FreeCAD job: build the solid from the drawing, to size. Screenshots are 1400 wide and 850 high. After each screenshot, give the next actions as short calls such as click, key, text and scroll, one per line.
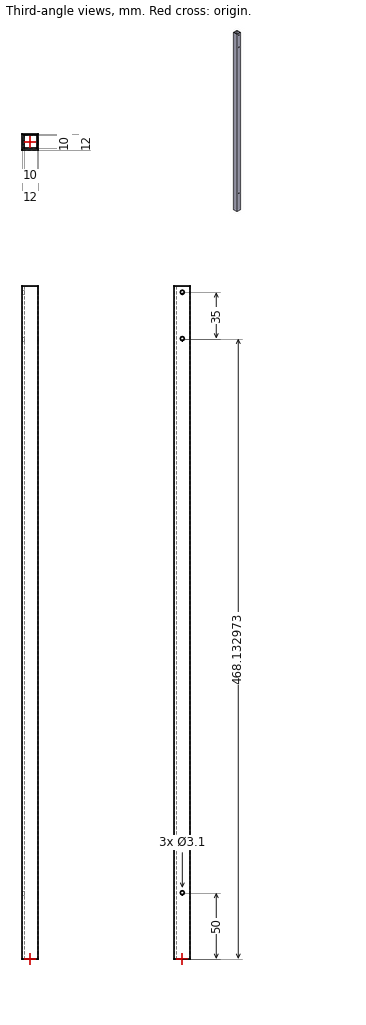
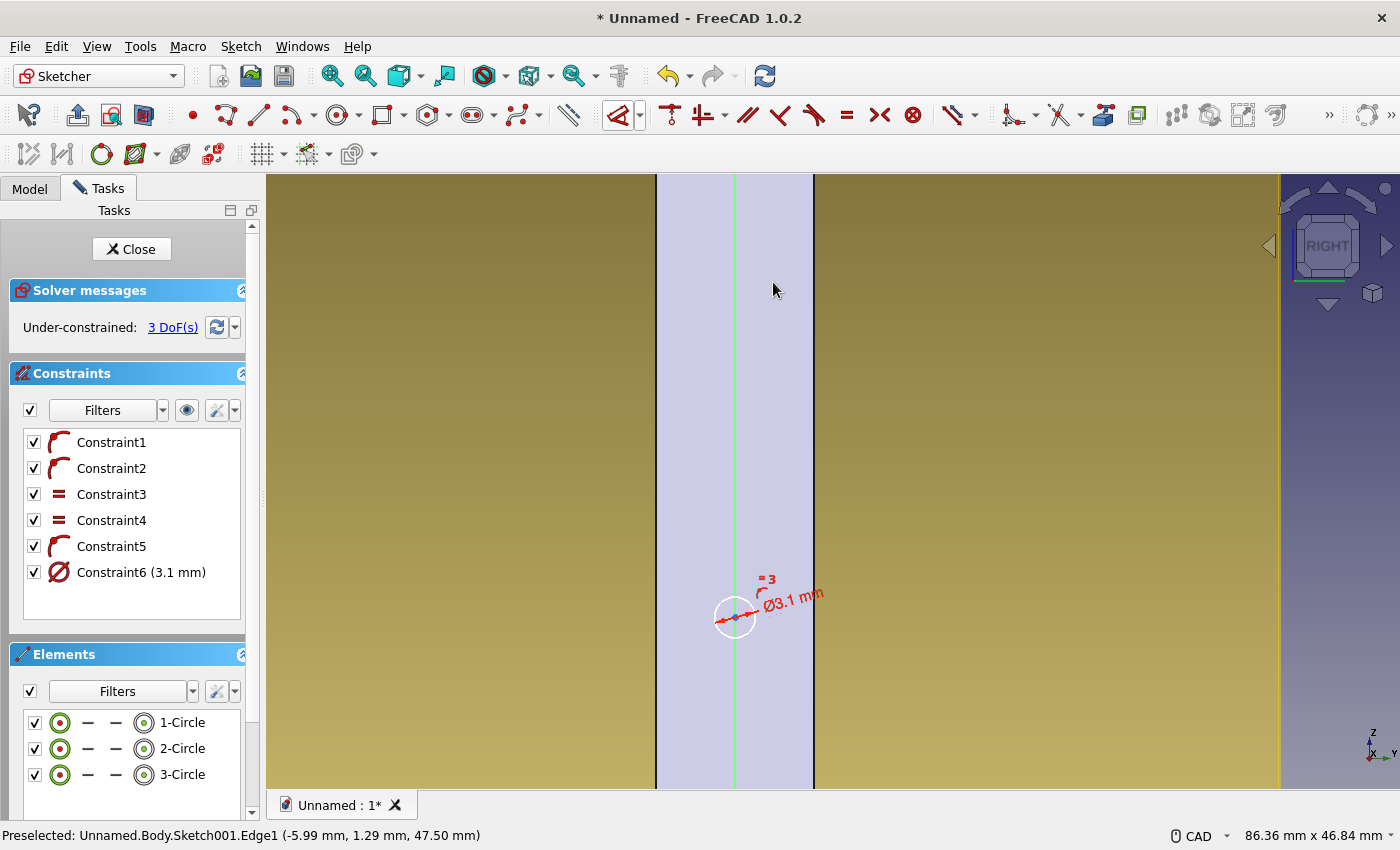
scroll(766, 646, down, 14)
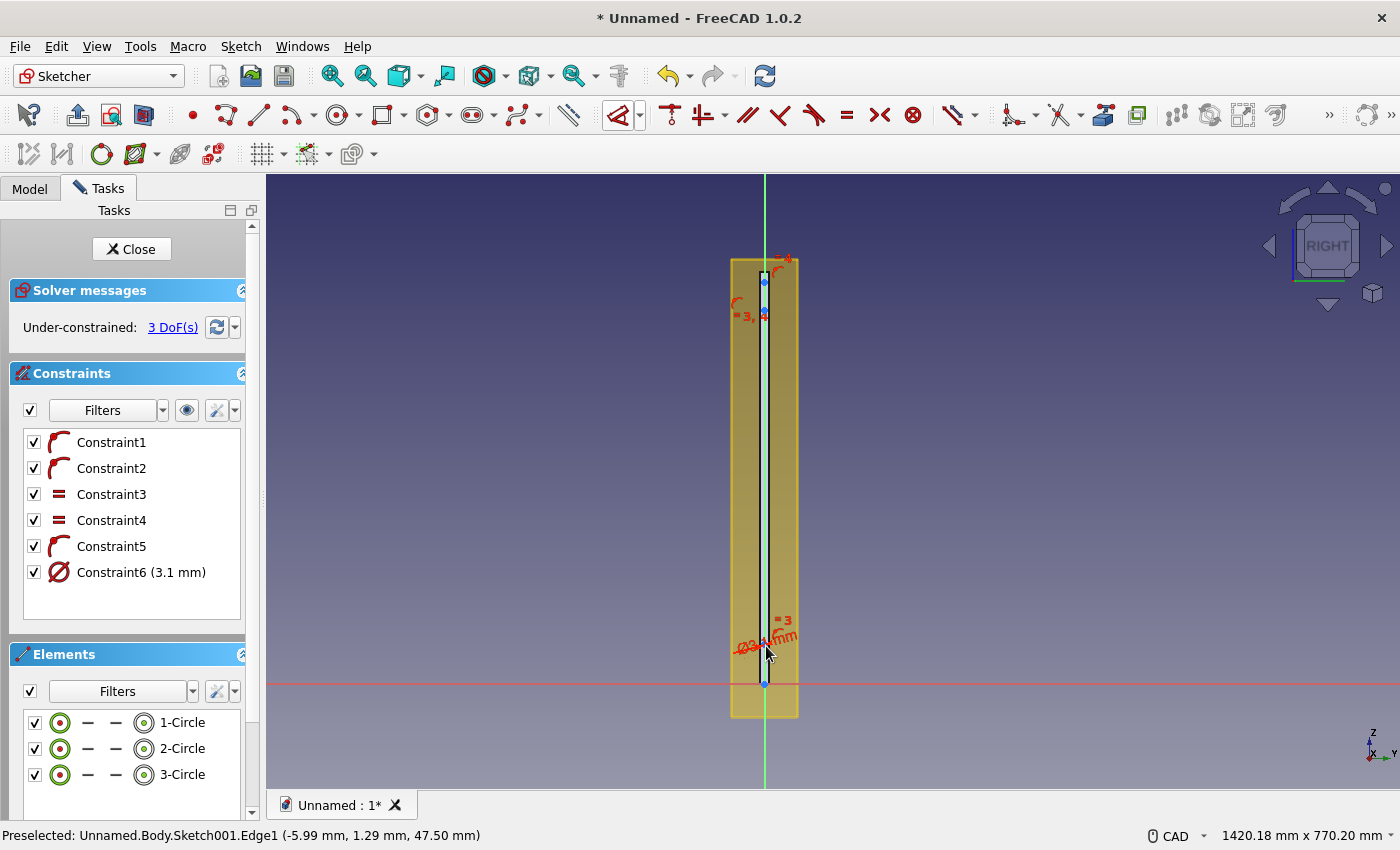
click(765, 645)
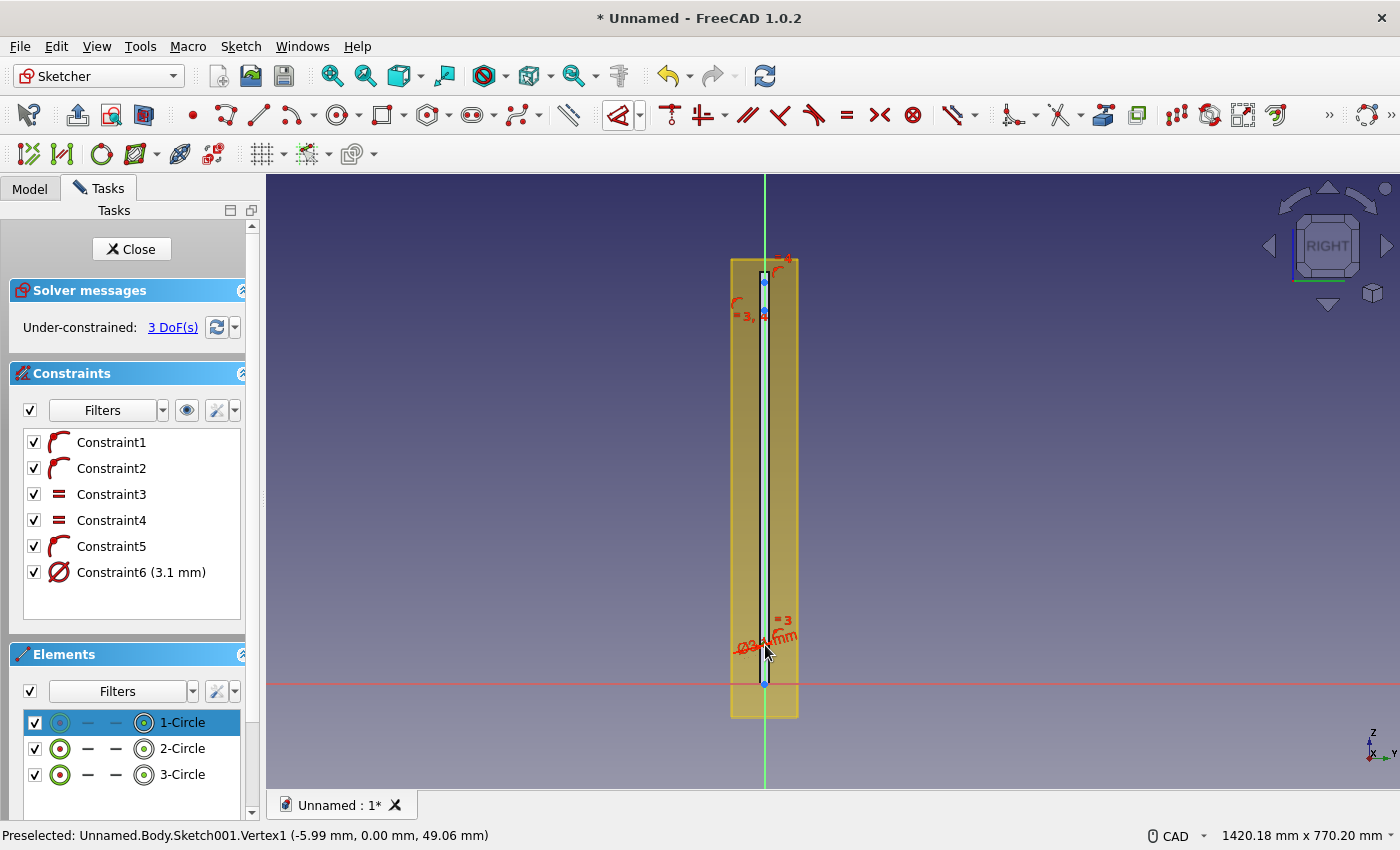
click(640, 116)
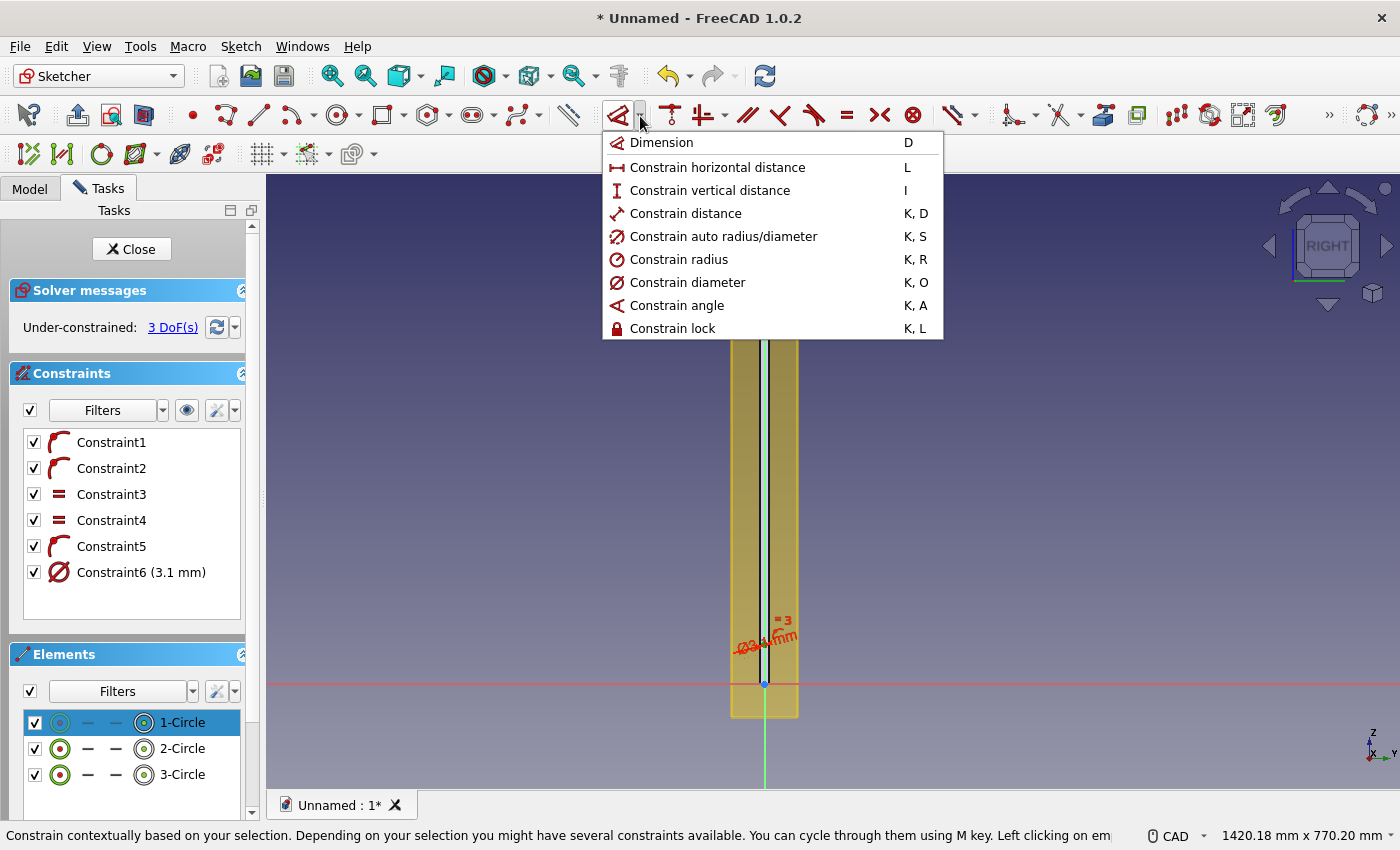
click(773, 190)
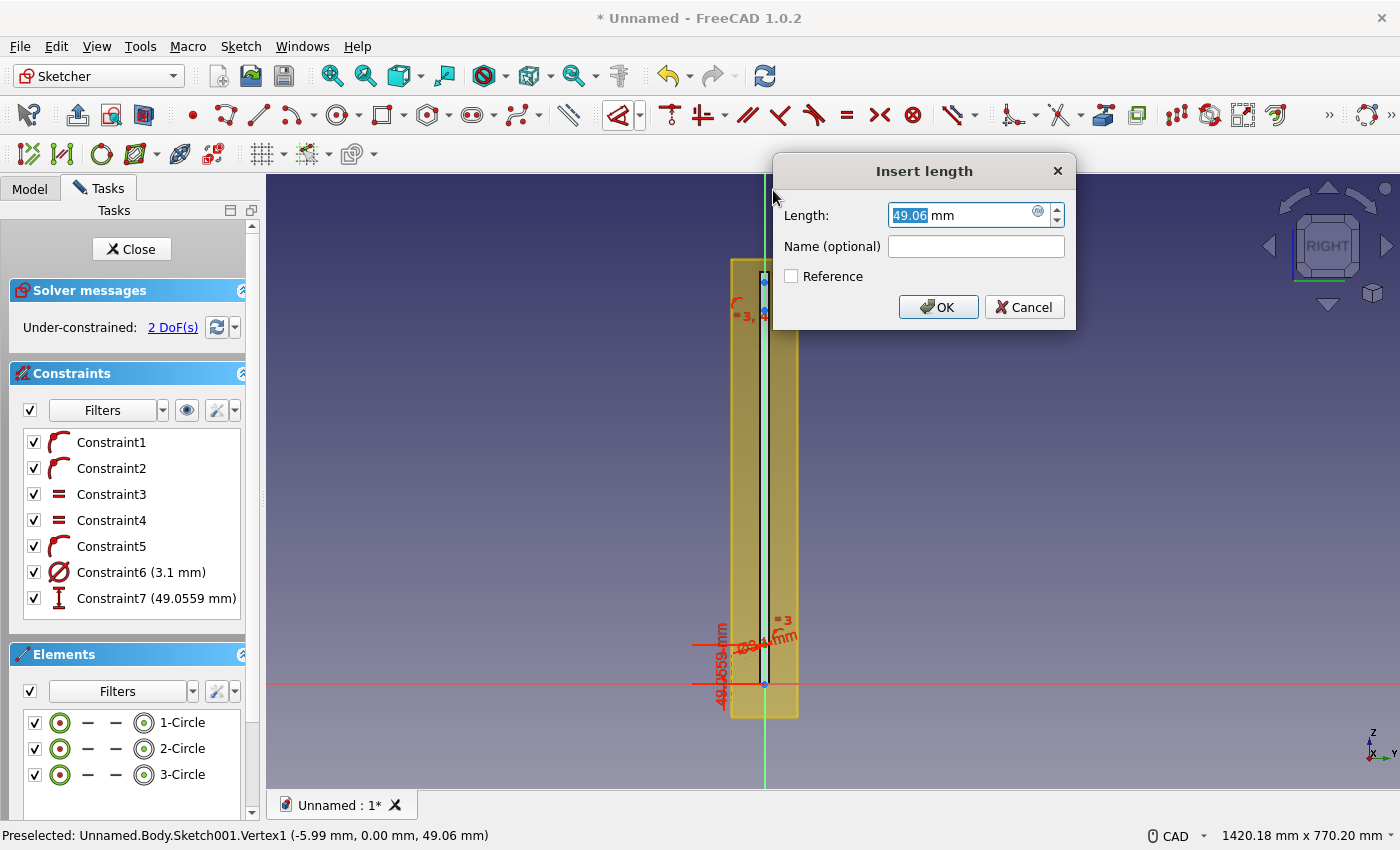
text(50)
key(Return)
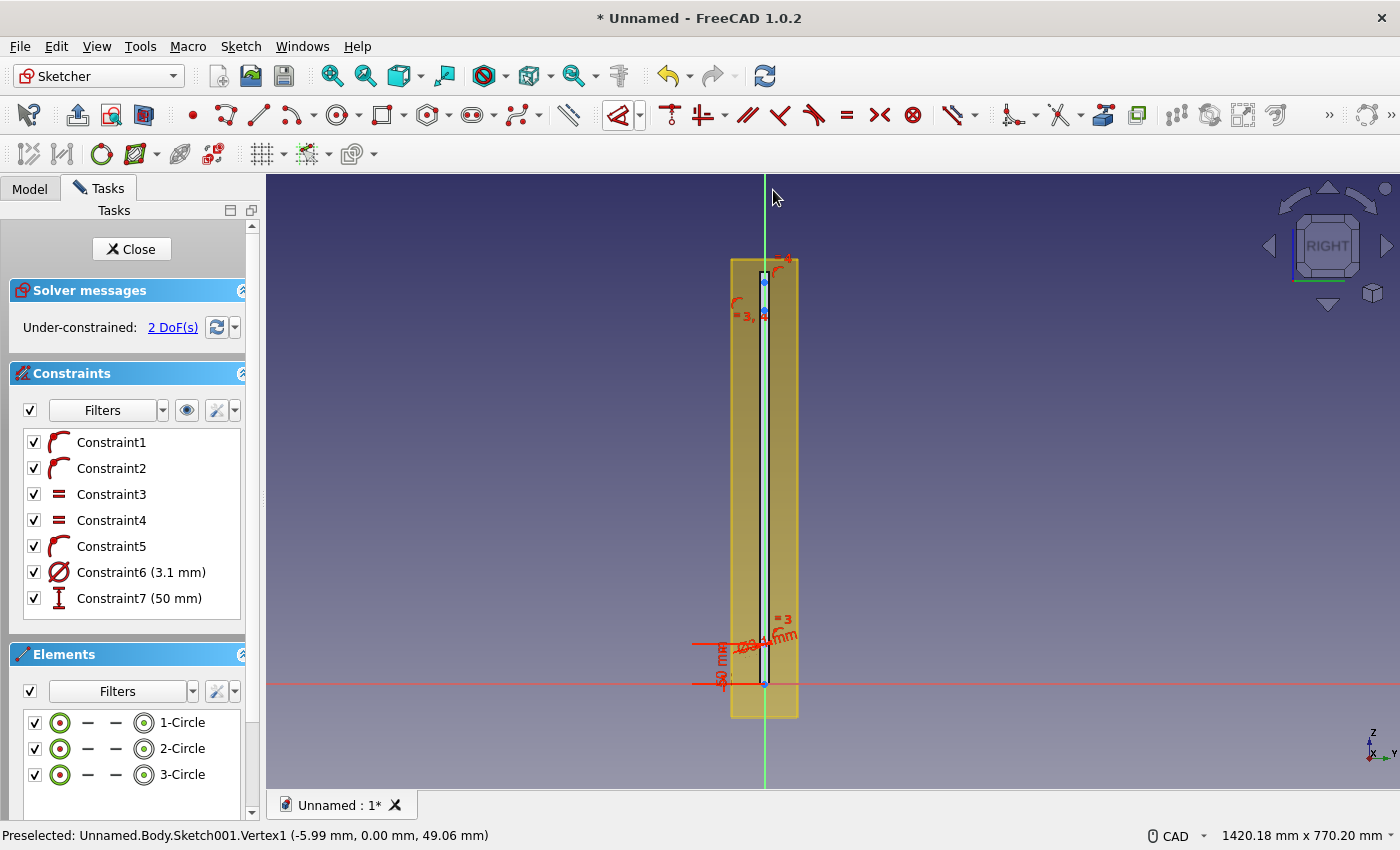
scroll(765, 311, up, 2)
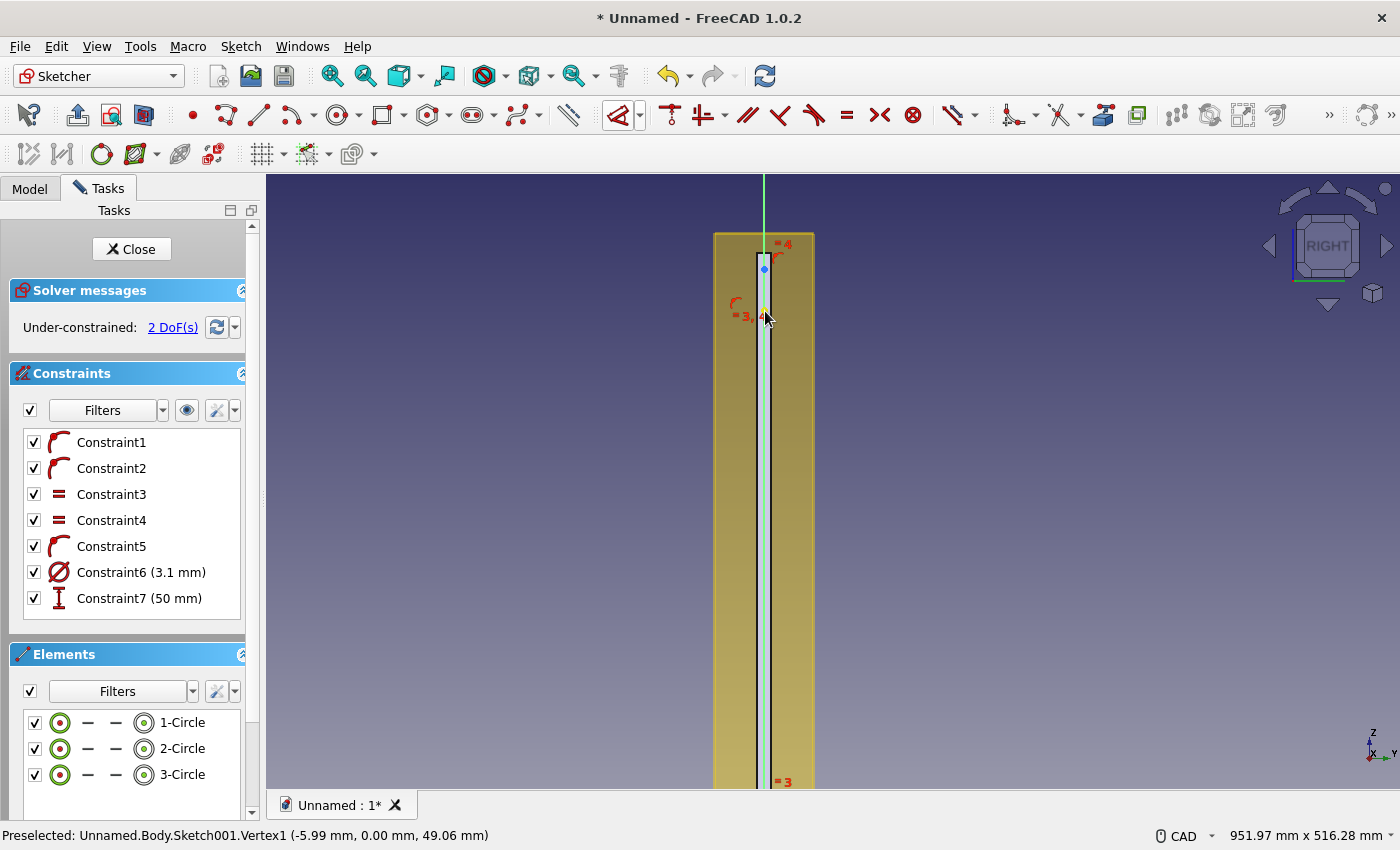
click(764, 311)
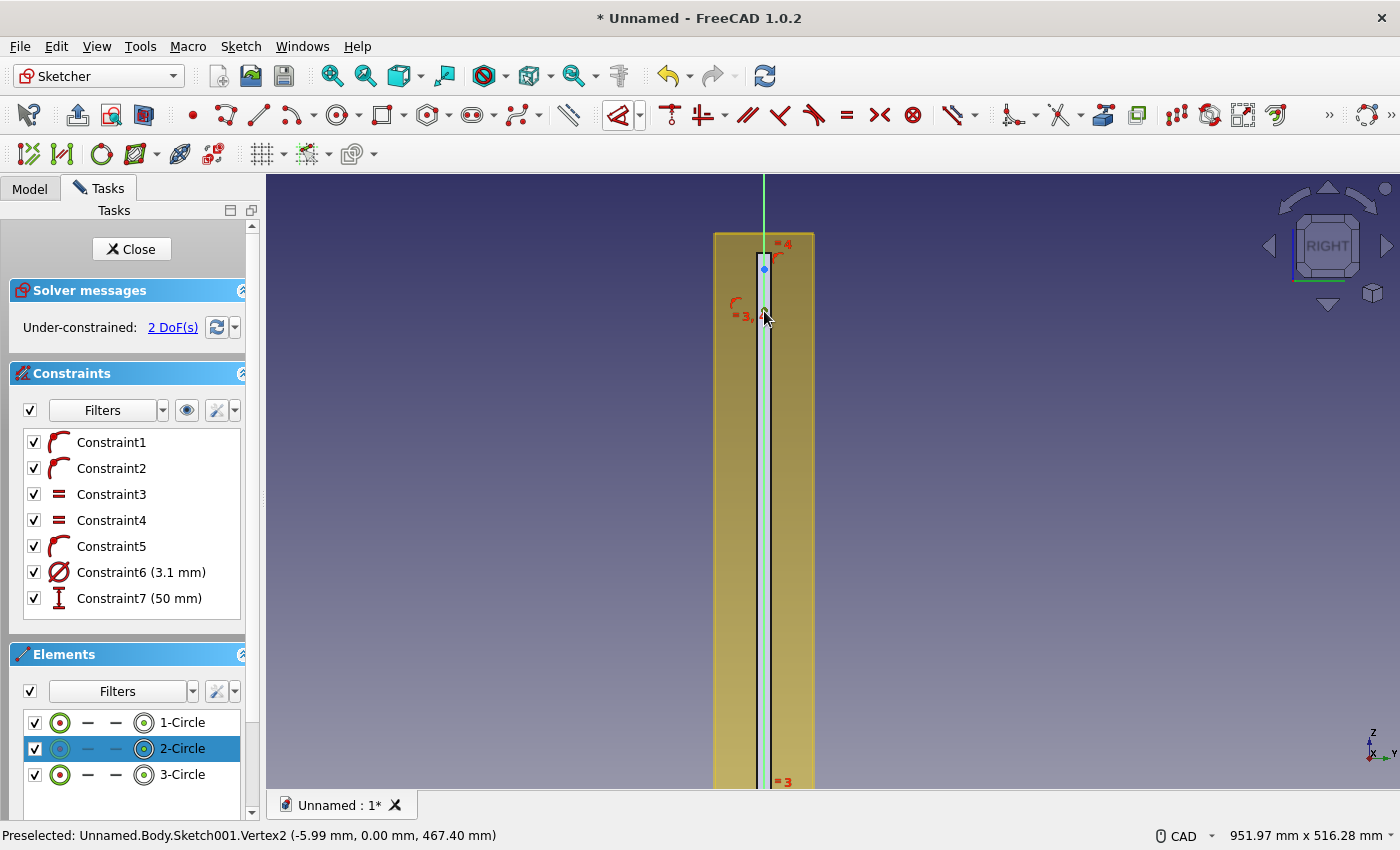
click(764, 269)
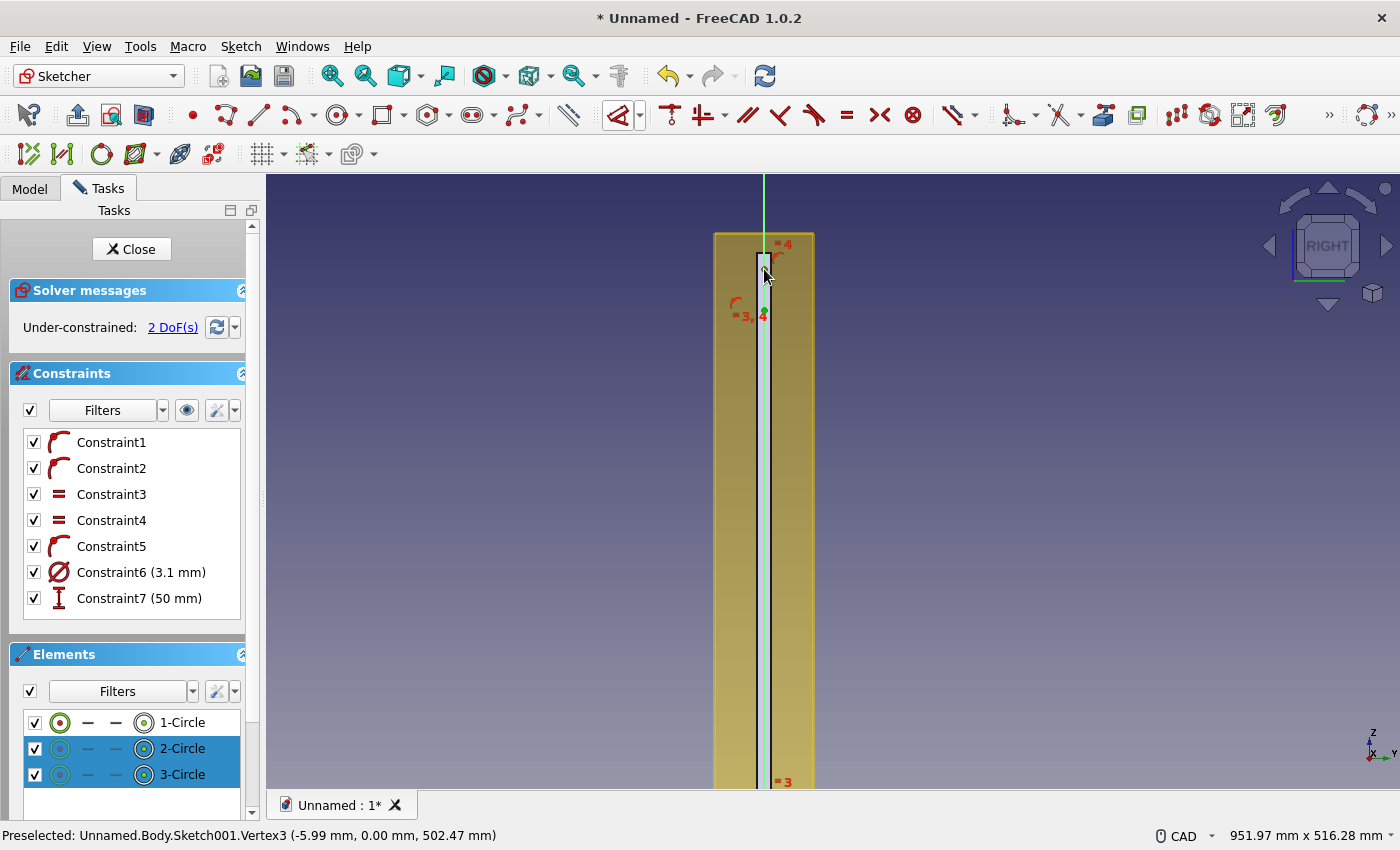
click(640, 116)